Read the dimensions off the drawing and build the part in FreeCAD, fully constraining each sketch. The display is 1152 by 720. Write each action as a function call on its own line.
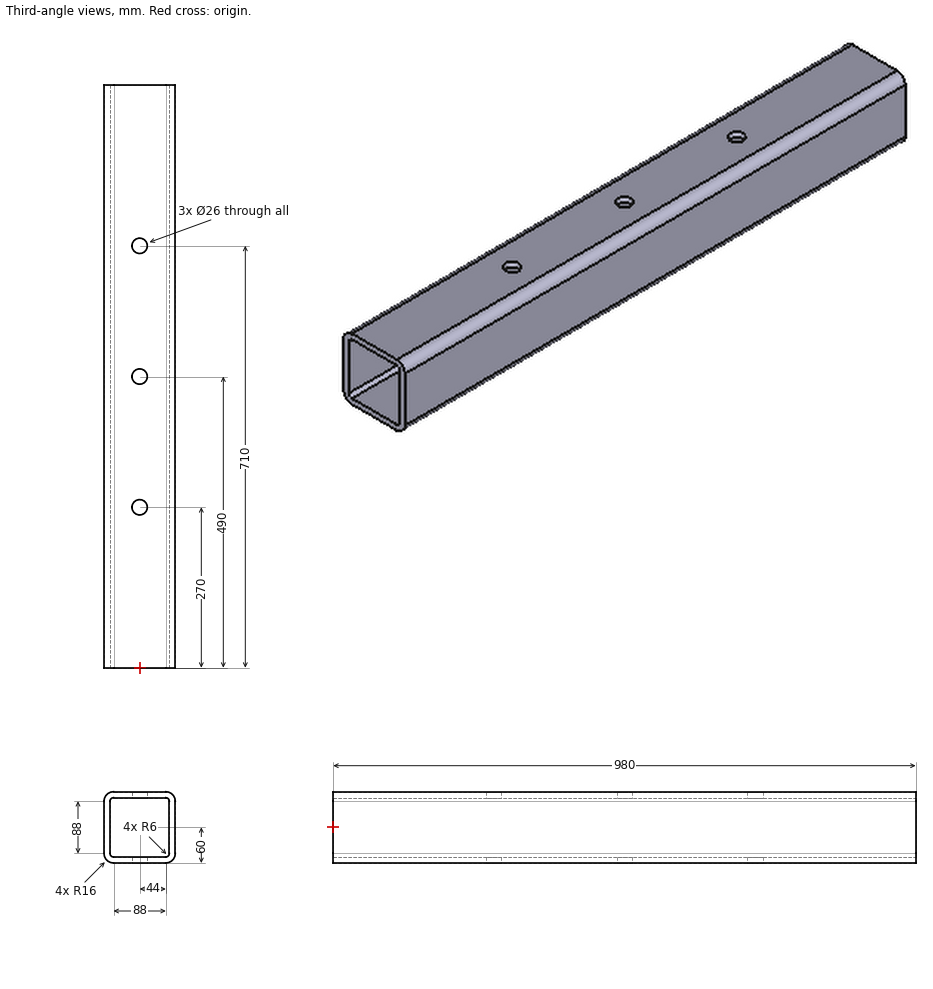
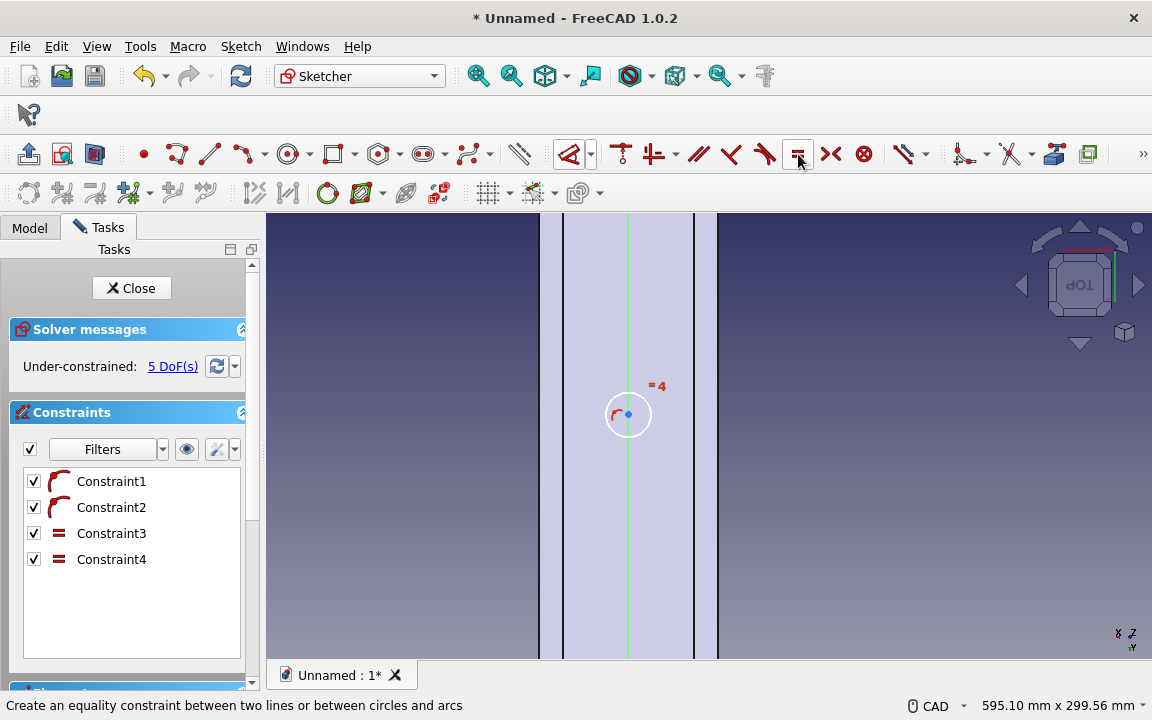
scroll(644, 400, down, 7)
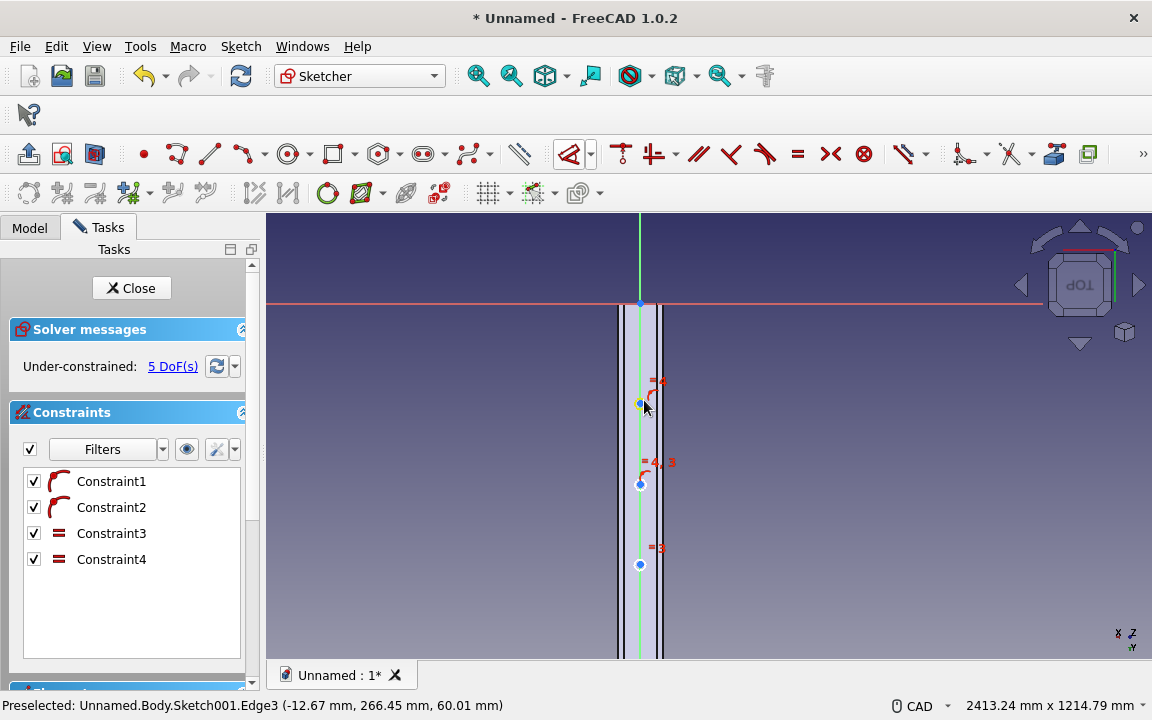
click(640, 565)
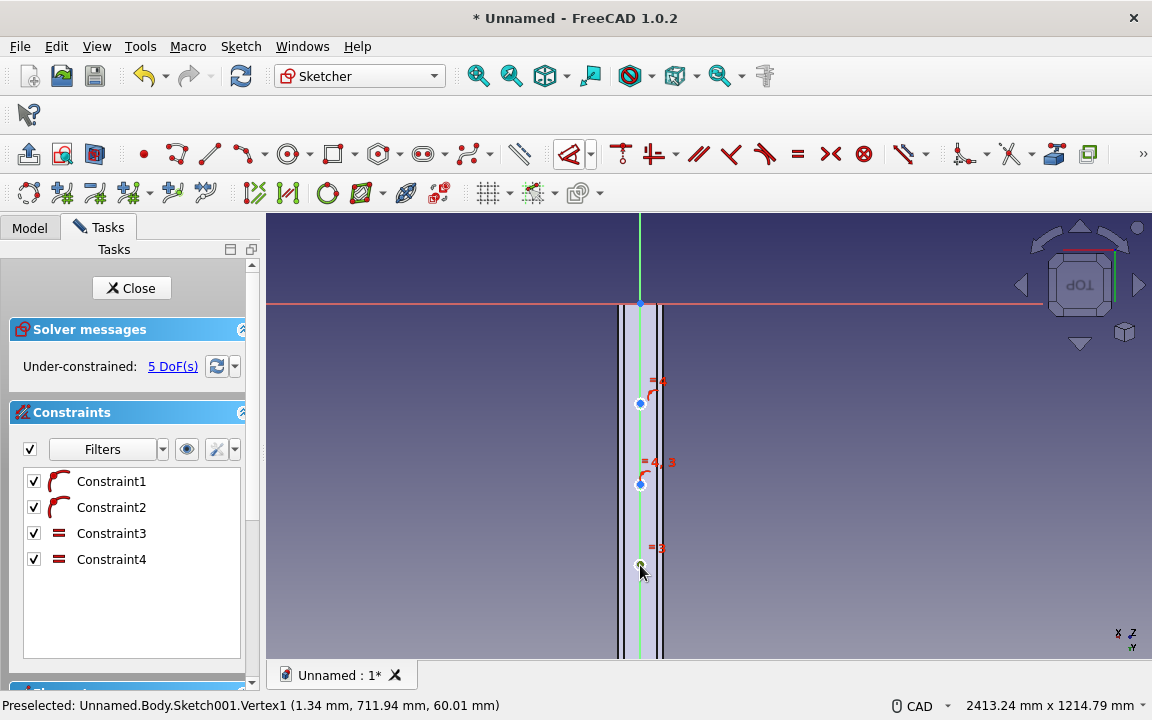
click(640, 603)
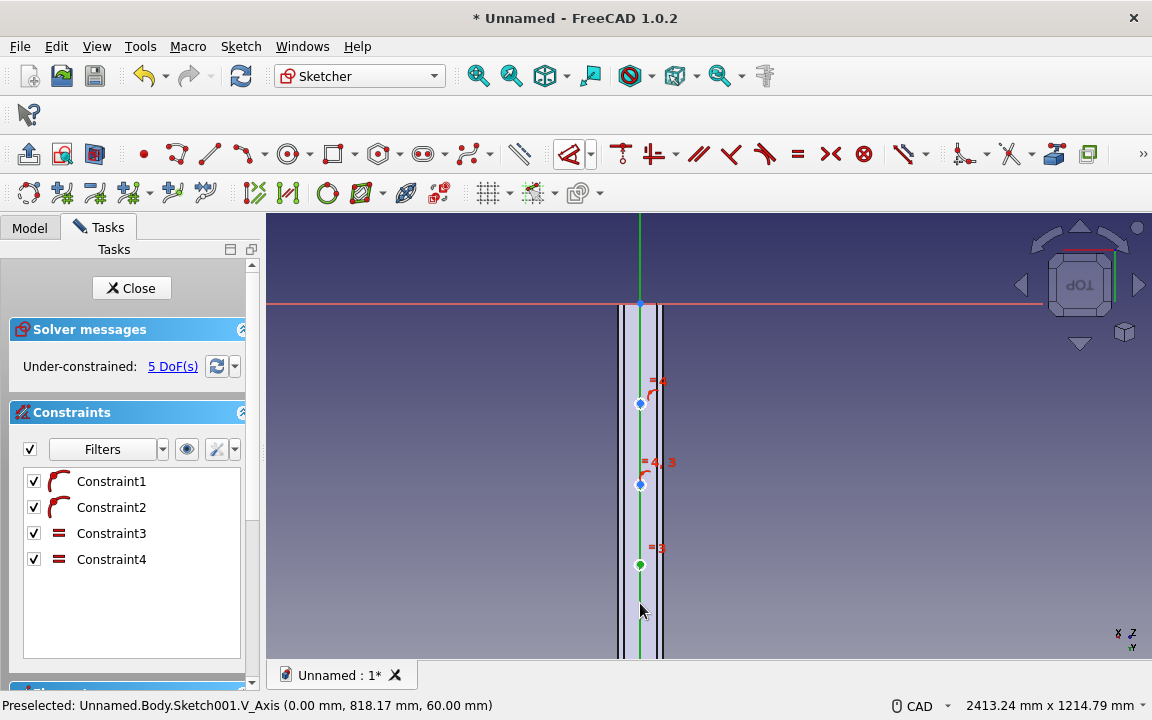
click(621, 154)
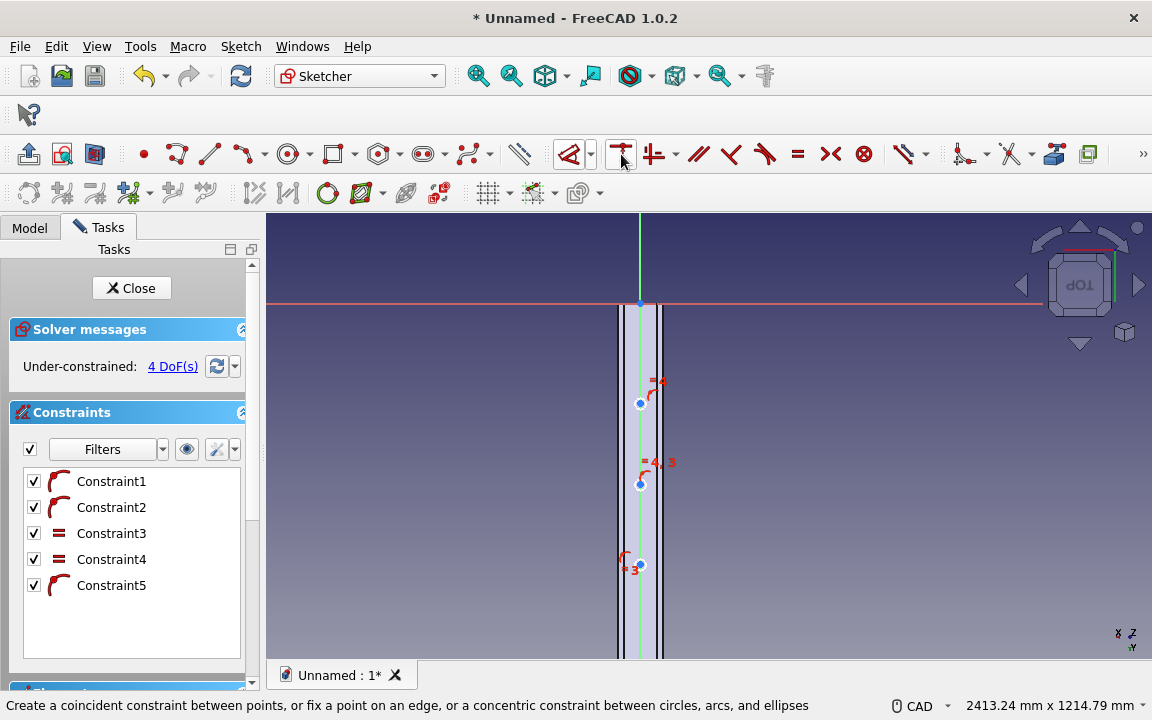
scroll(637, 561, up, 8)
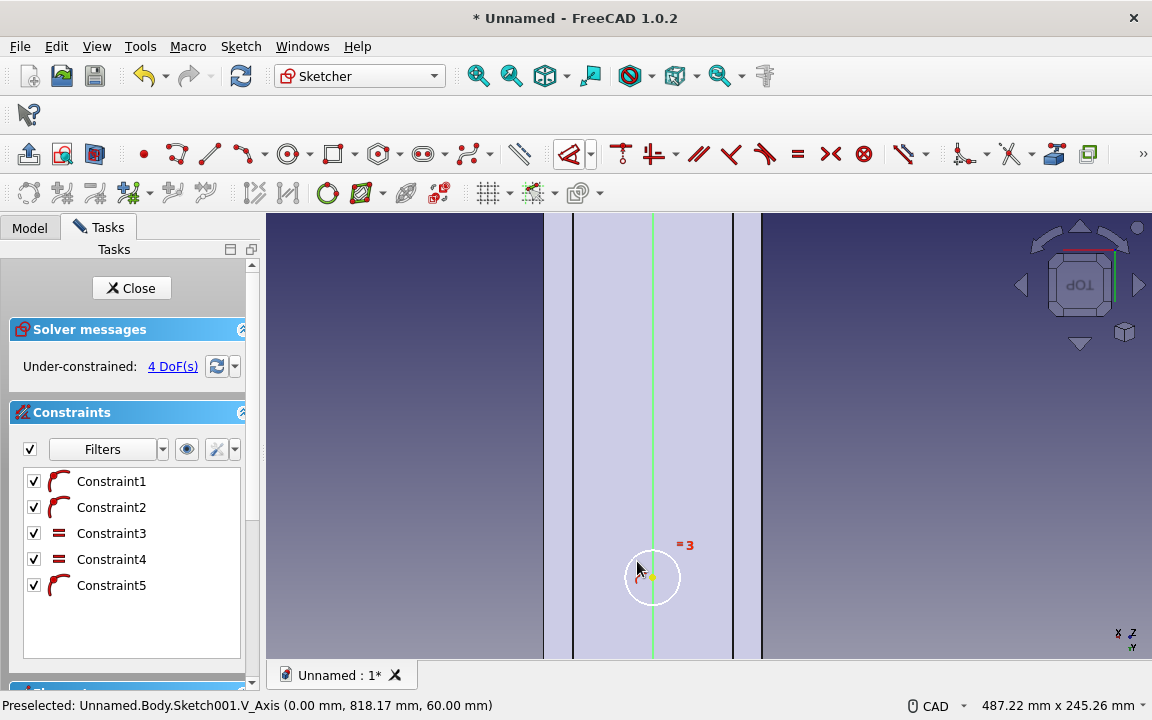
click(633, 558)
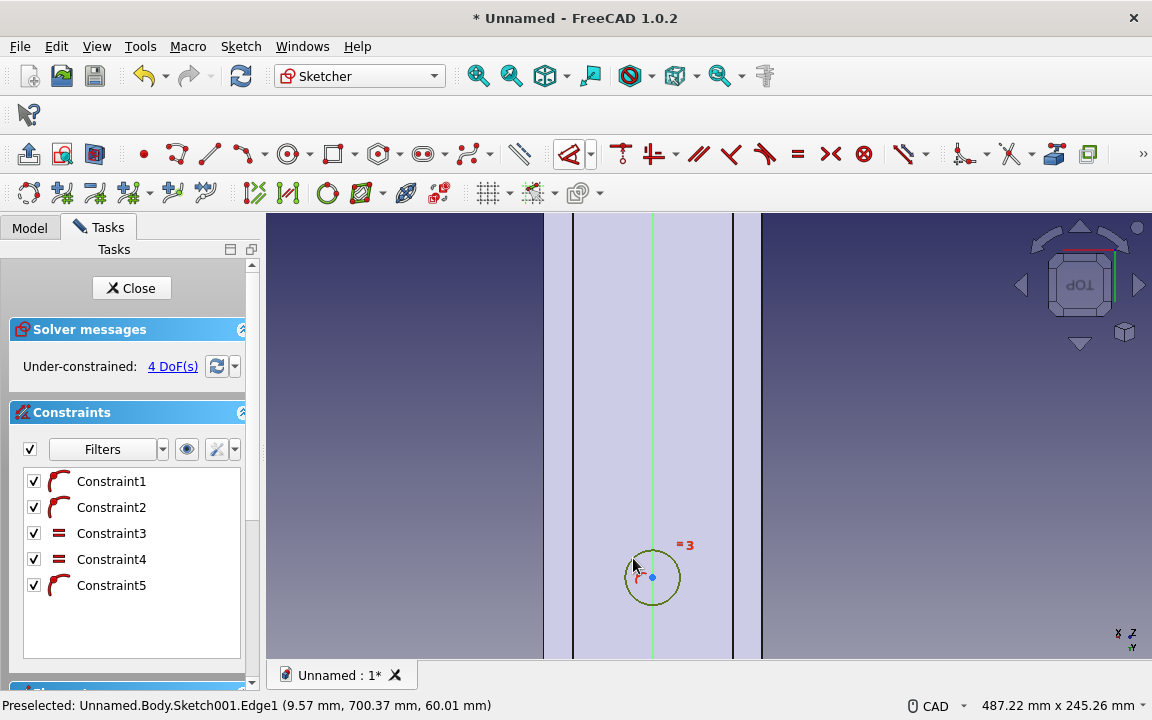
key(k)
key(o)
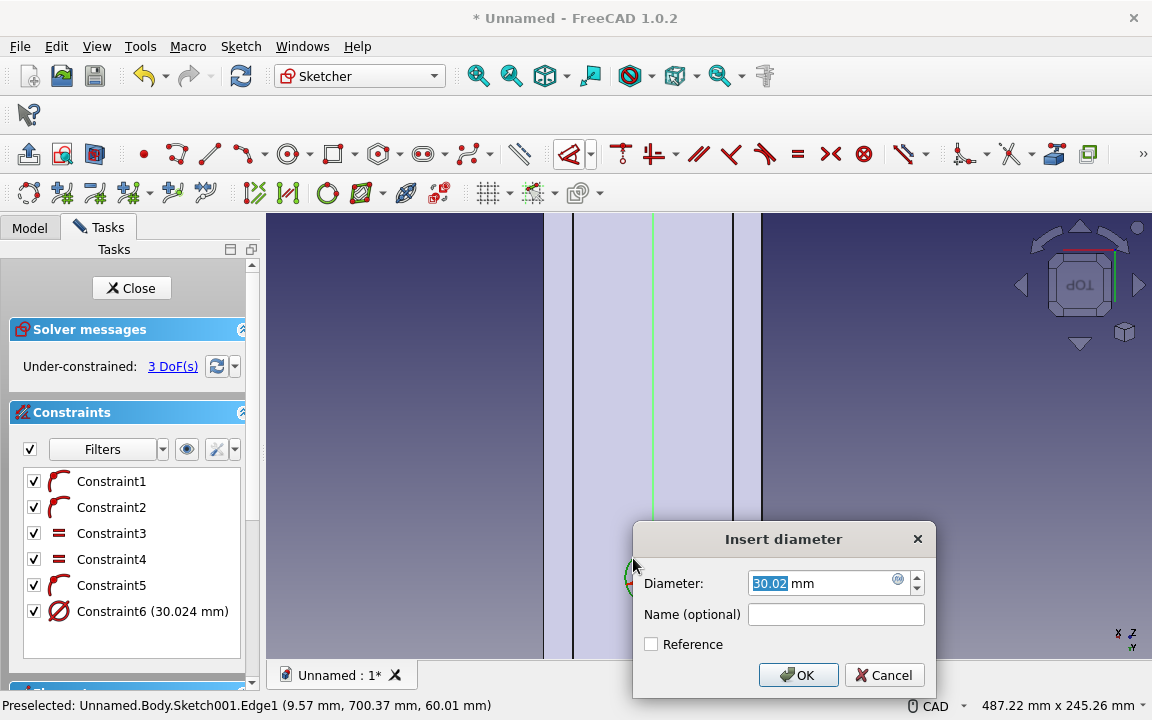
text(26)
key(Return)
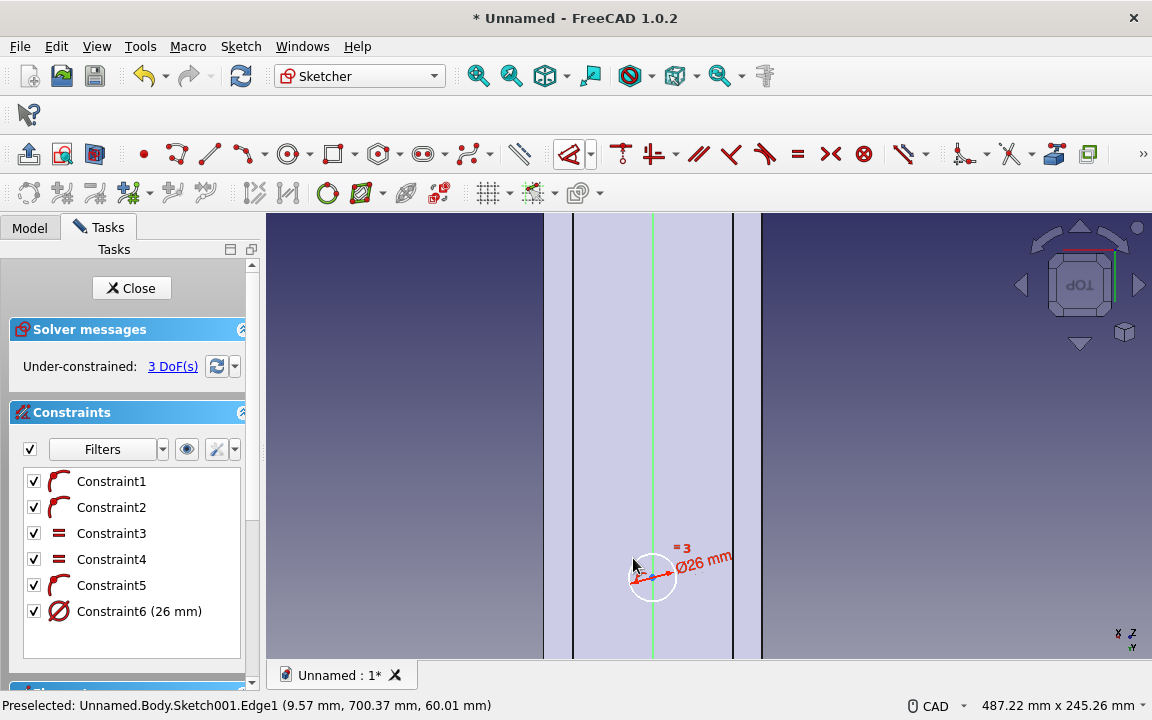
scroll(637, 561, down, 8)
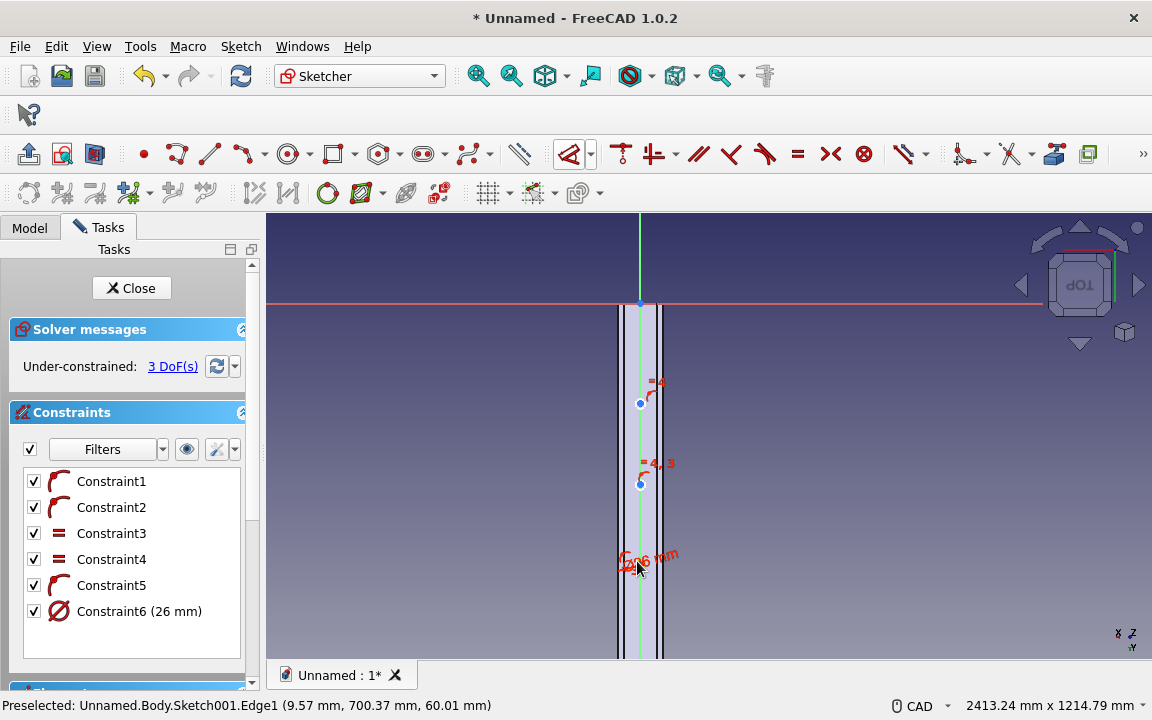
click(640, 565)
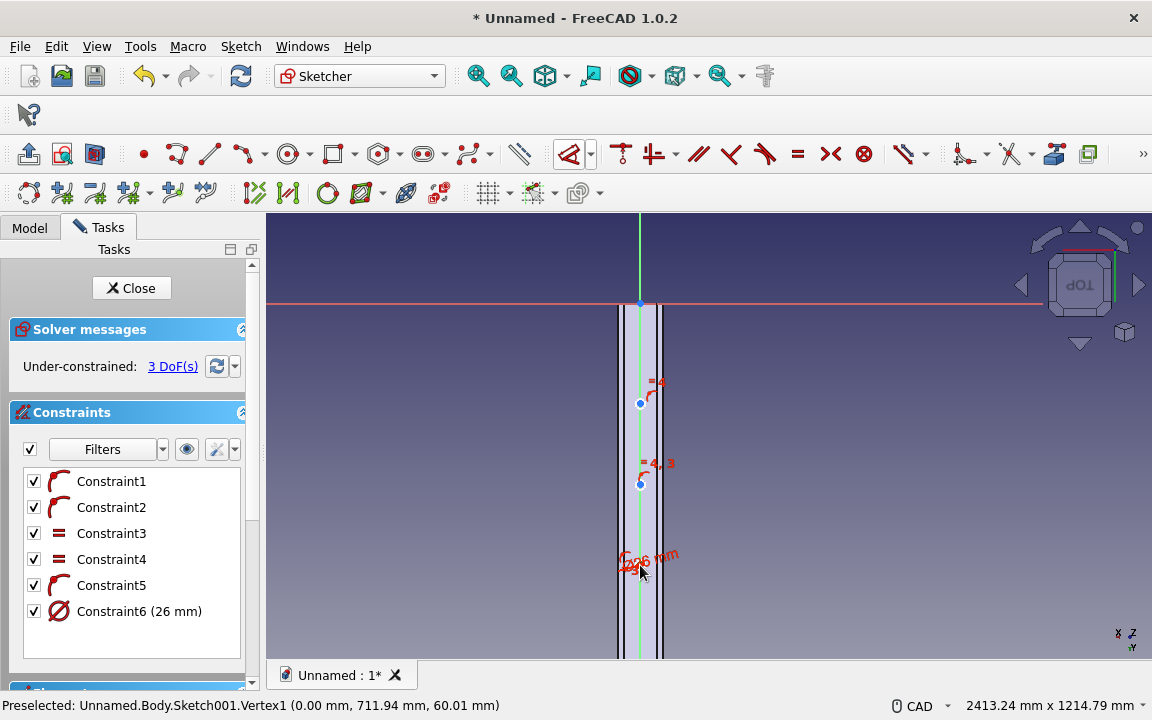
key(i)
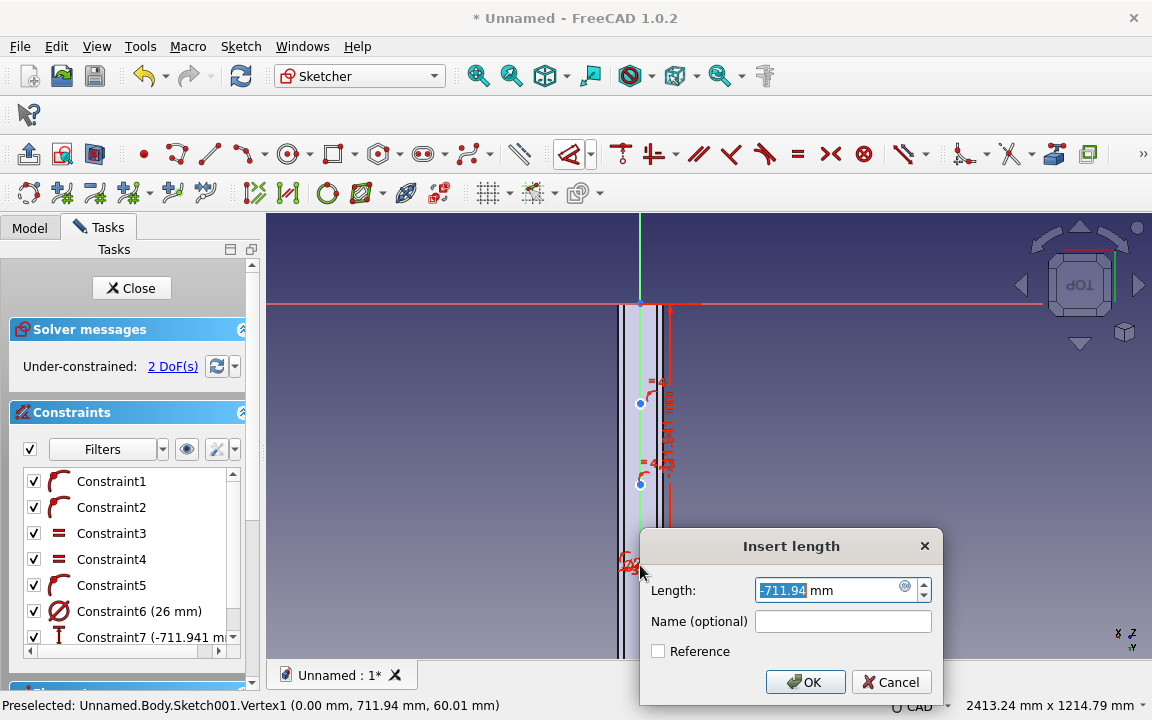
text(-710)
key(Return)